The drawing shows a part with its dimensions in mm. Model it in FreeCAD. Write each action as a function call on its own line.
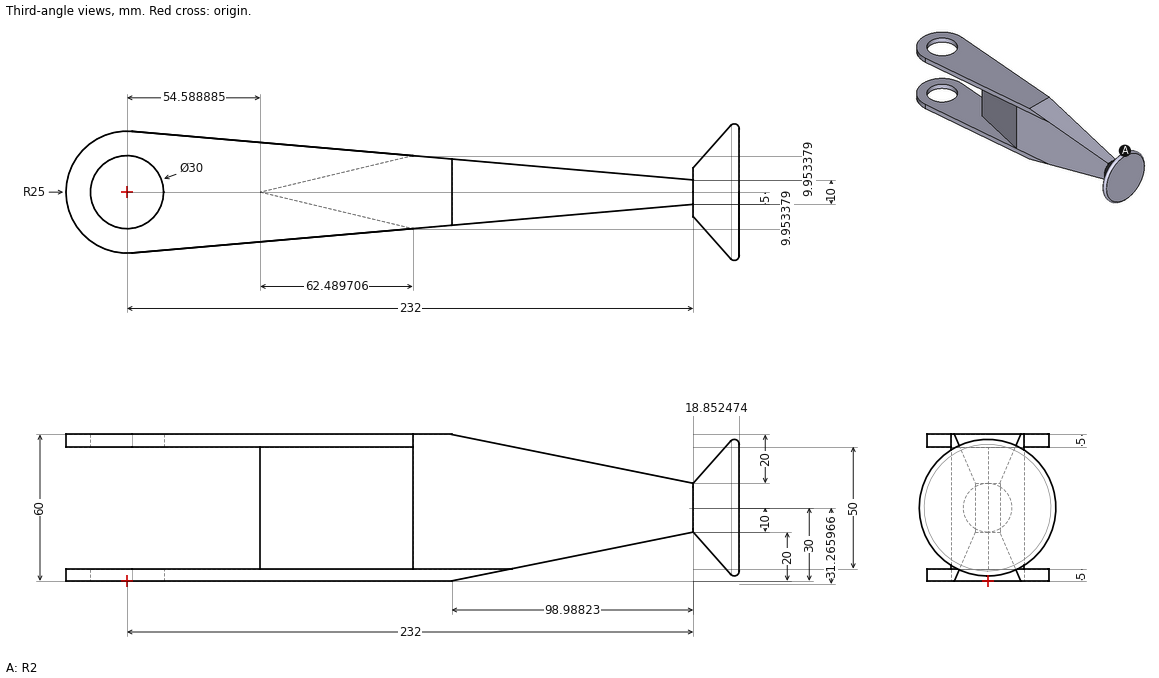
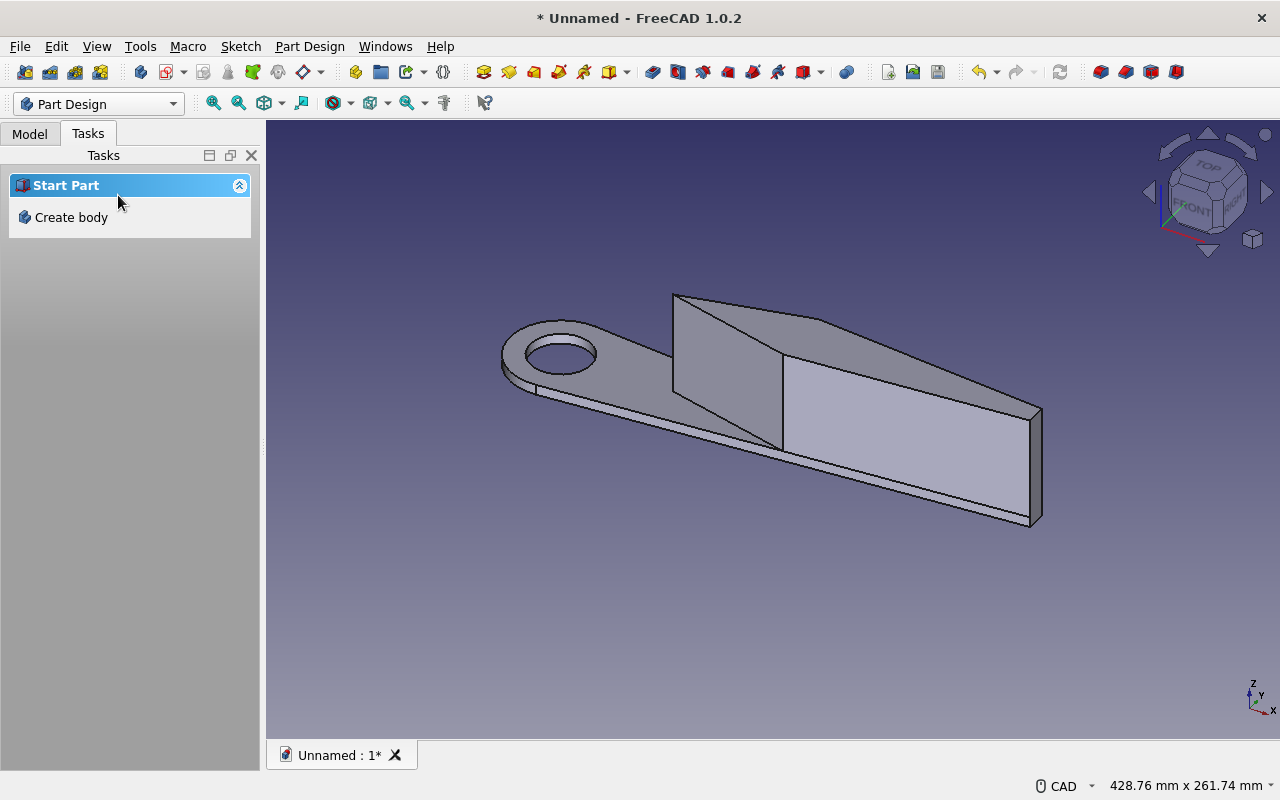
click(802, 336)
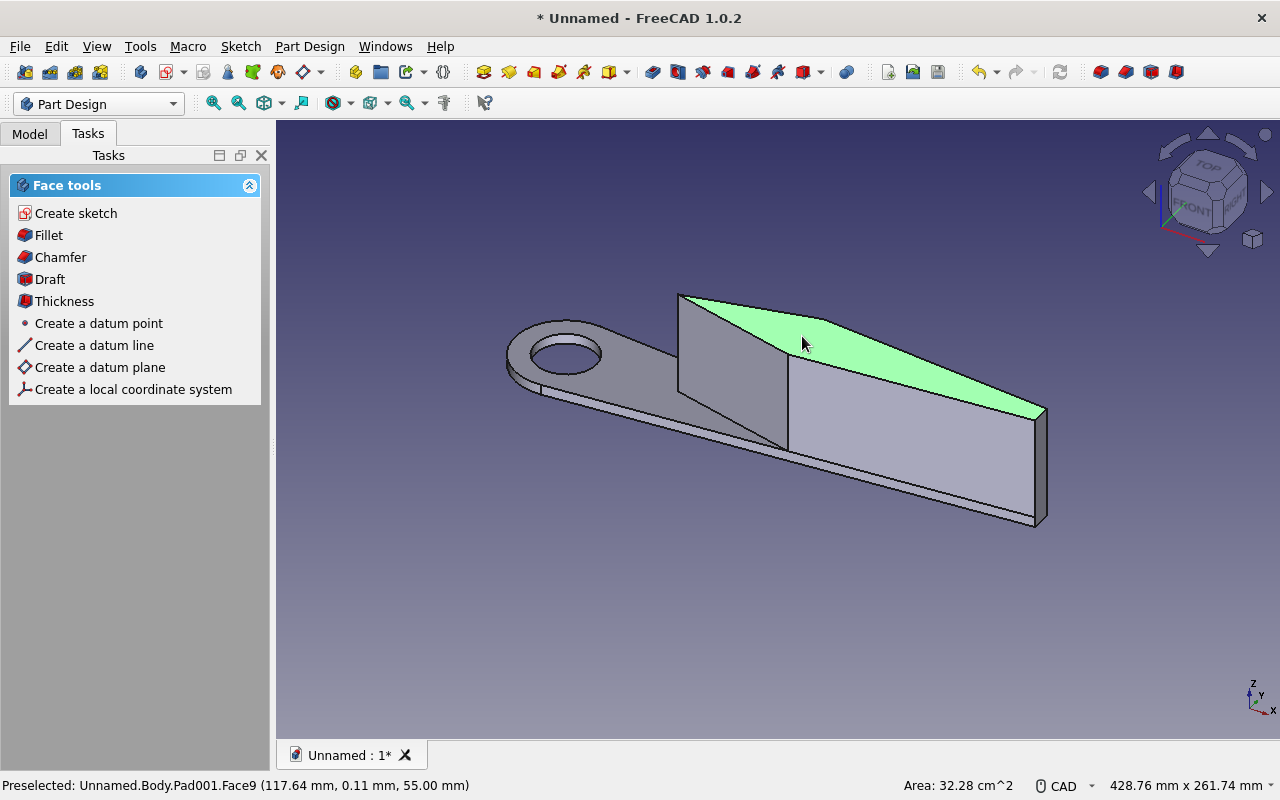
click(166, 72)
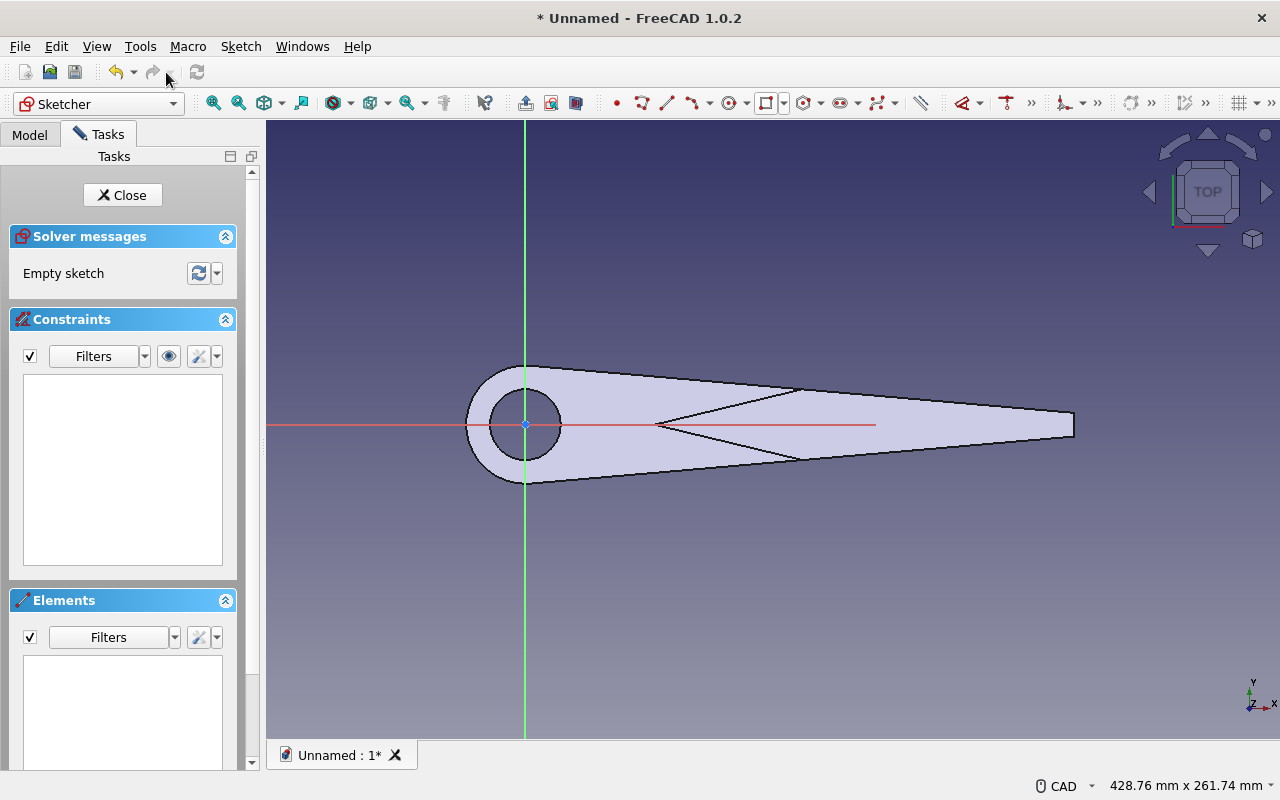
click(642, 104)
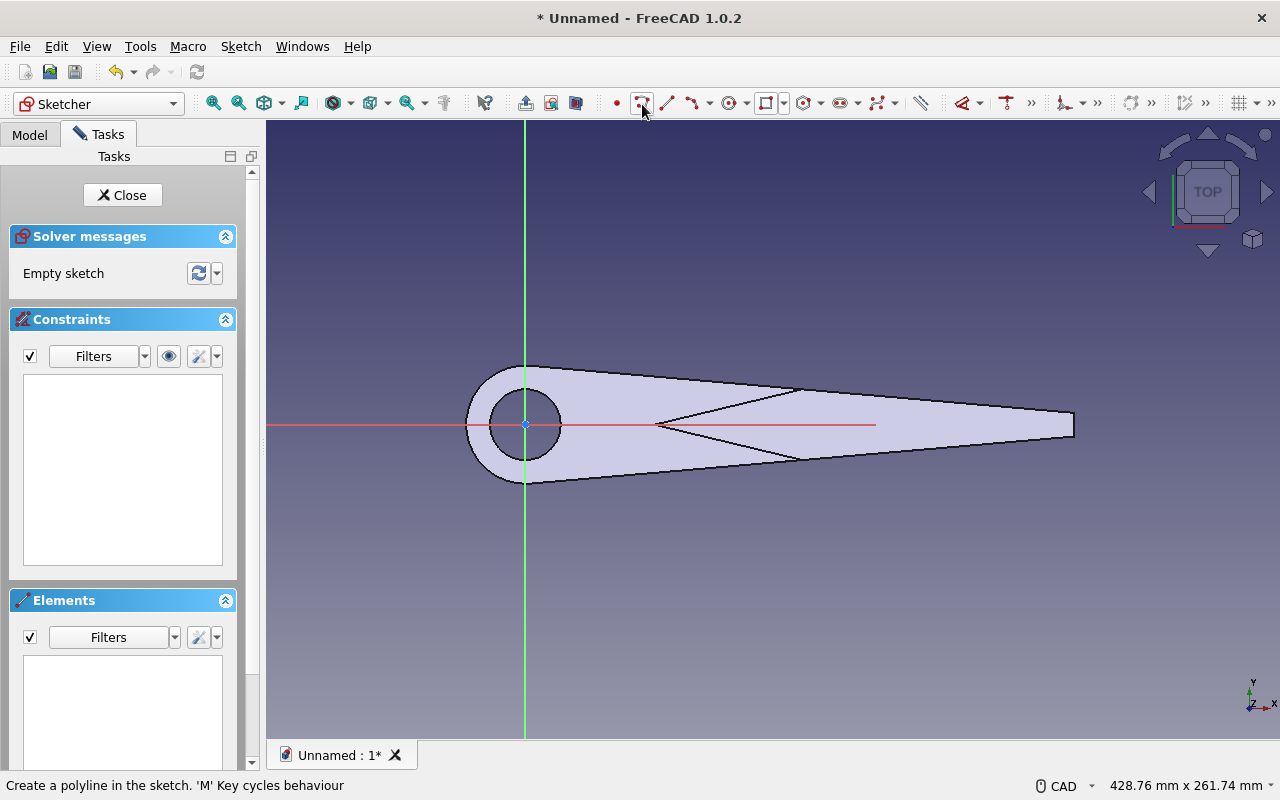
scroll(530, 484, up, 6)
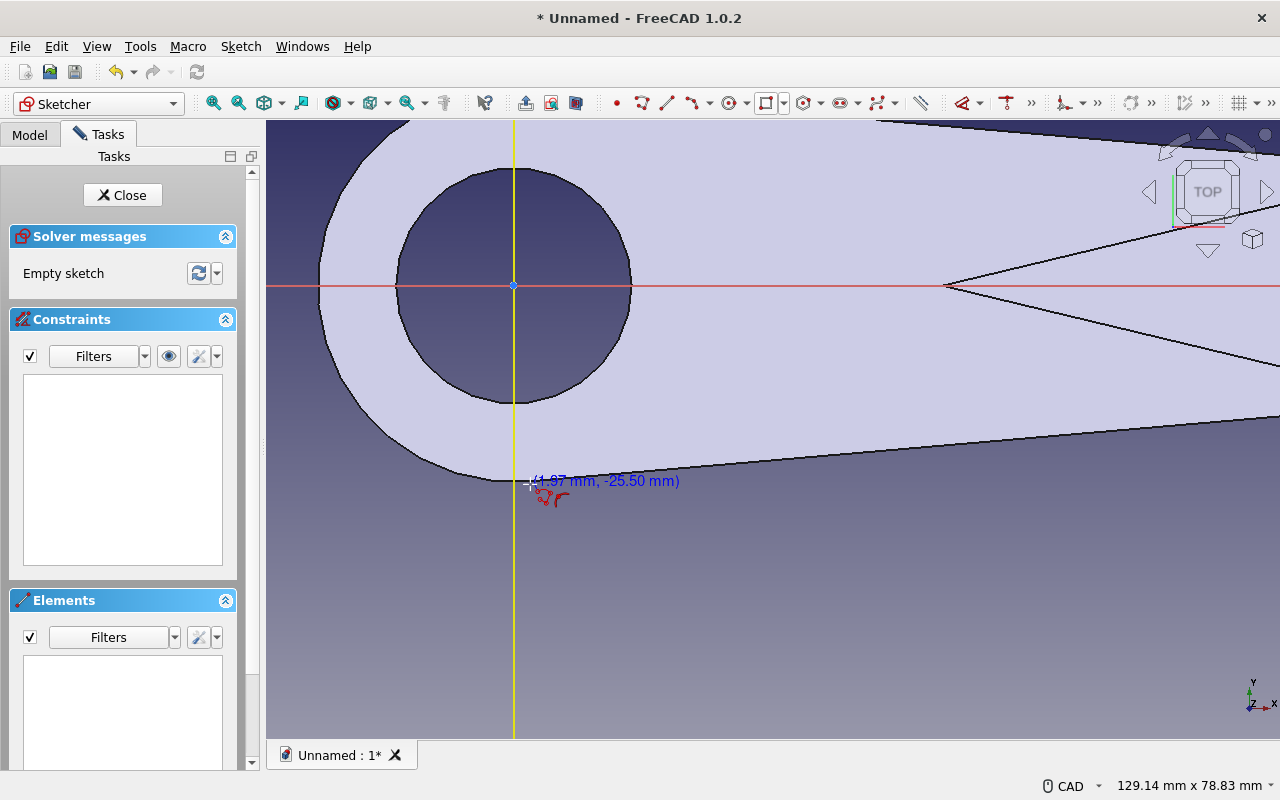
click(531, 481)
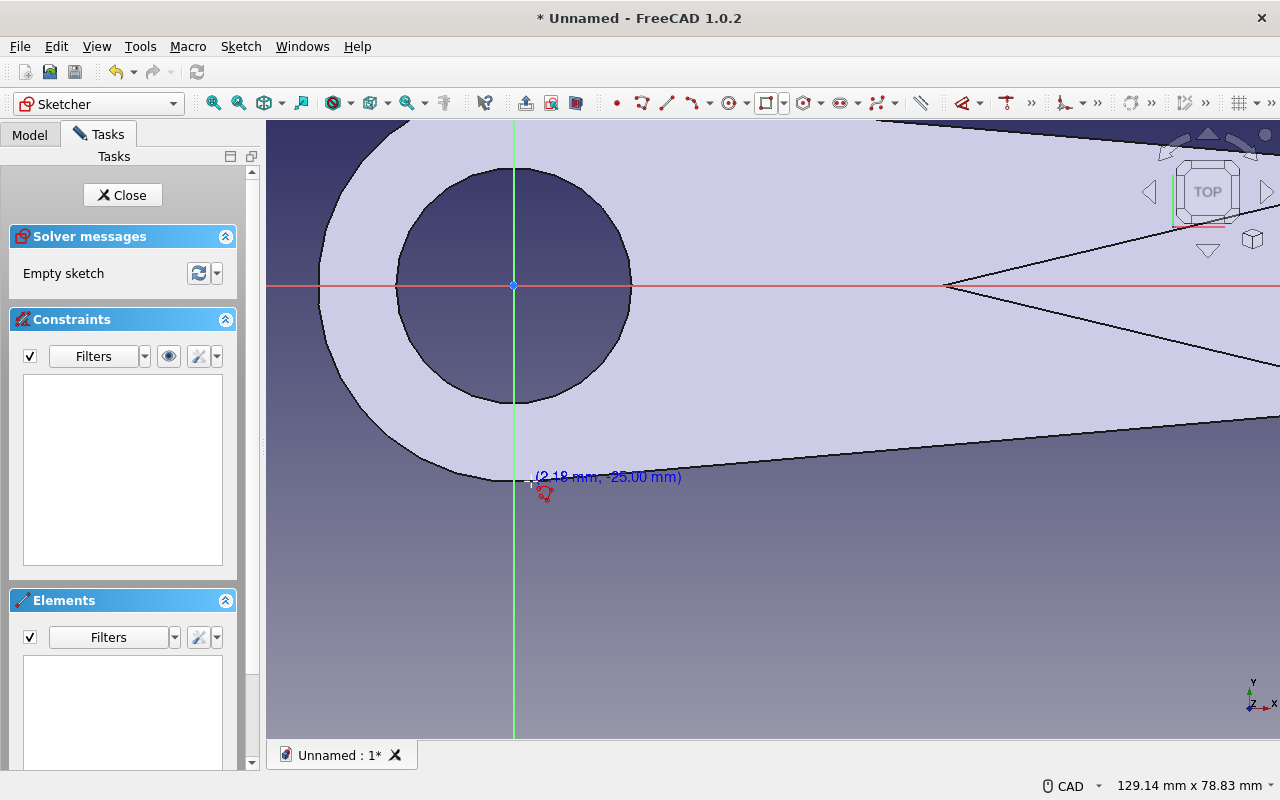
scroll(436, 491, down, 6)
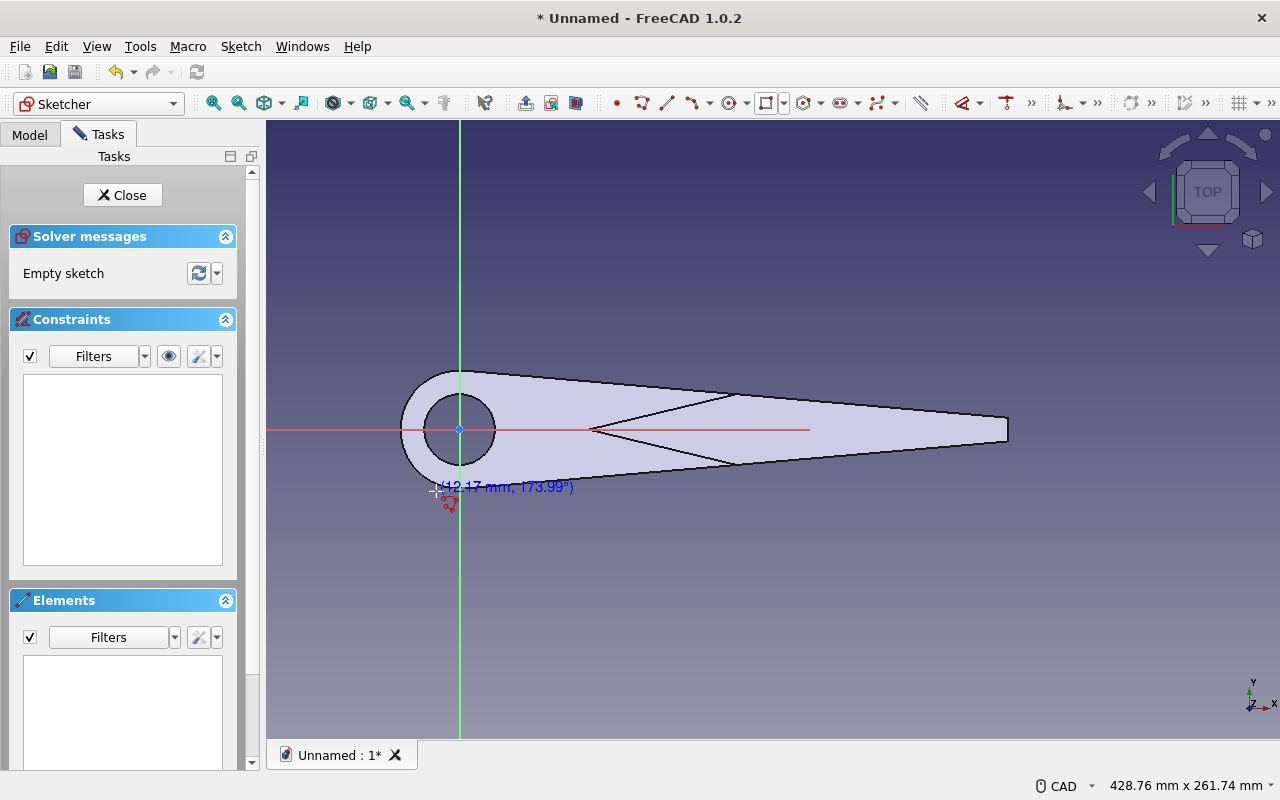
scroll(1008, 441, up, 2)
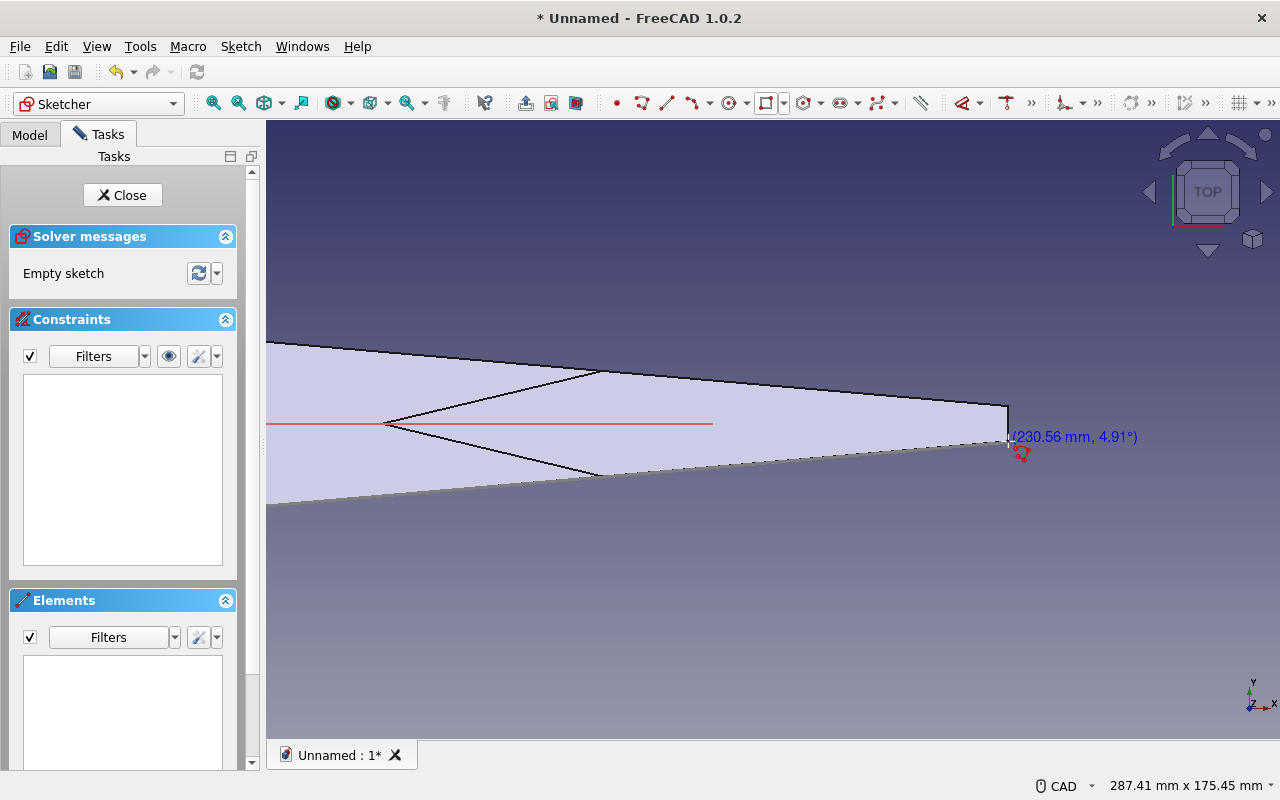
click(1008, 441)
click(1008, 406)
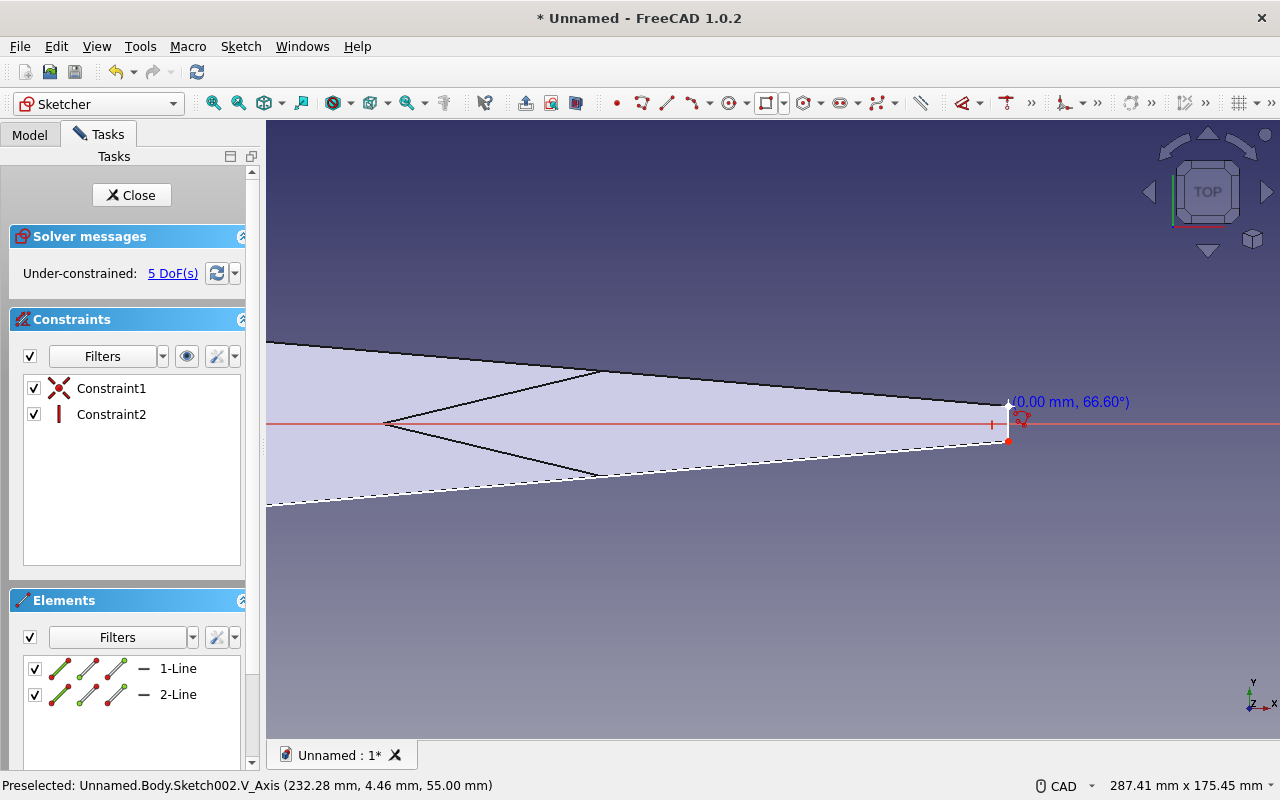
scroll(1009, 441, down, 2)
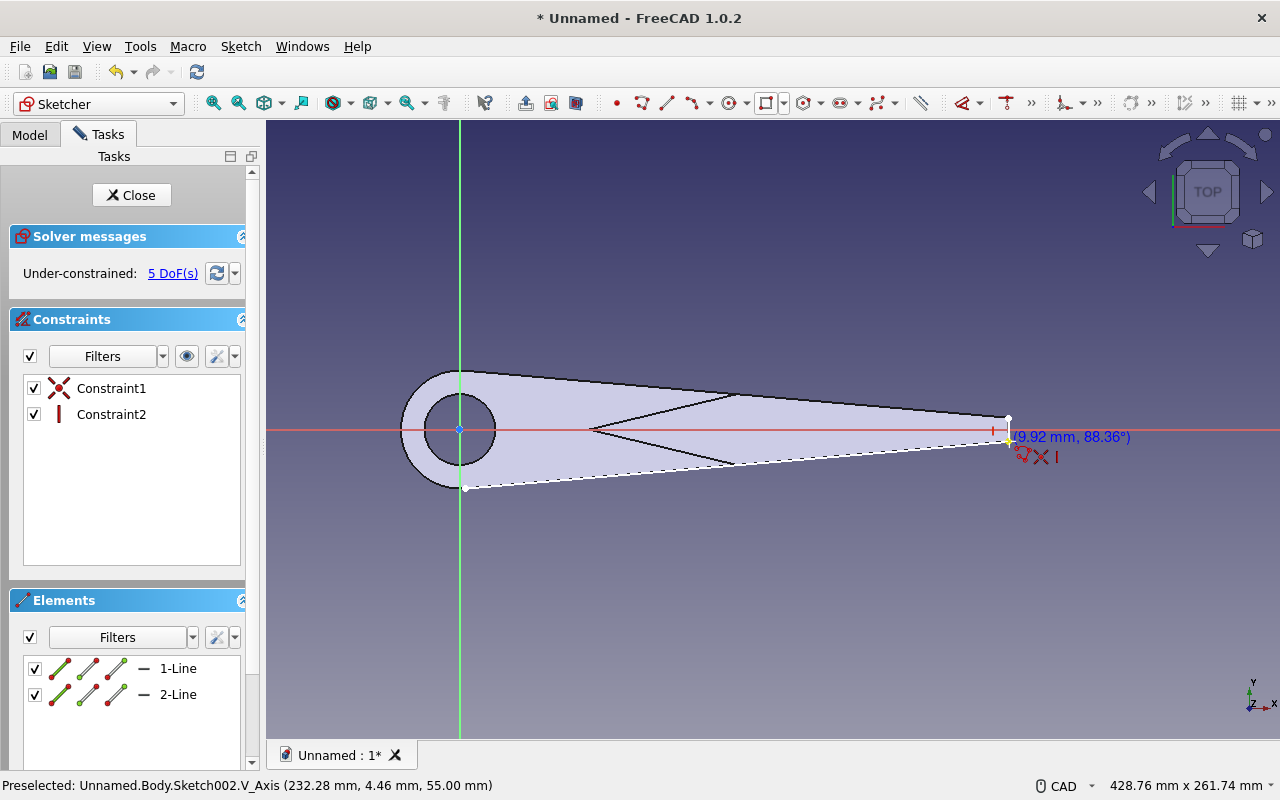
scroll(465, 371, up, 6)